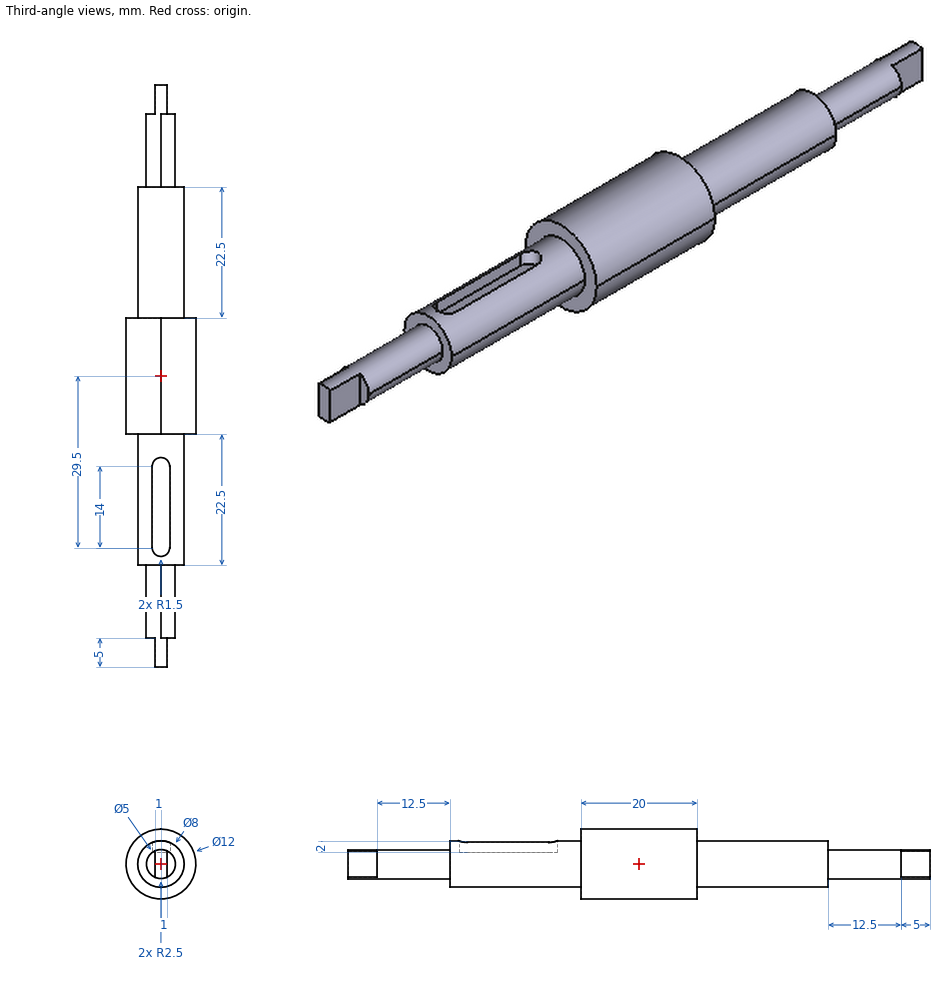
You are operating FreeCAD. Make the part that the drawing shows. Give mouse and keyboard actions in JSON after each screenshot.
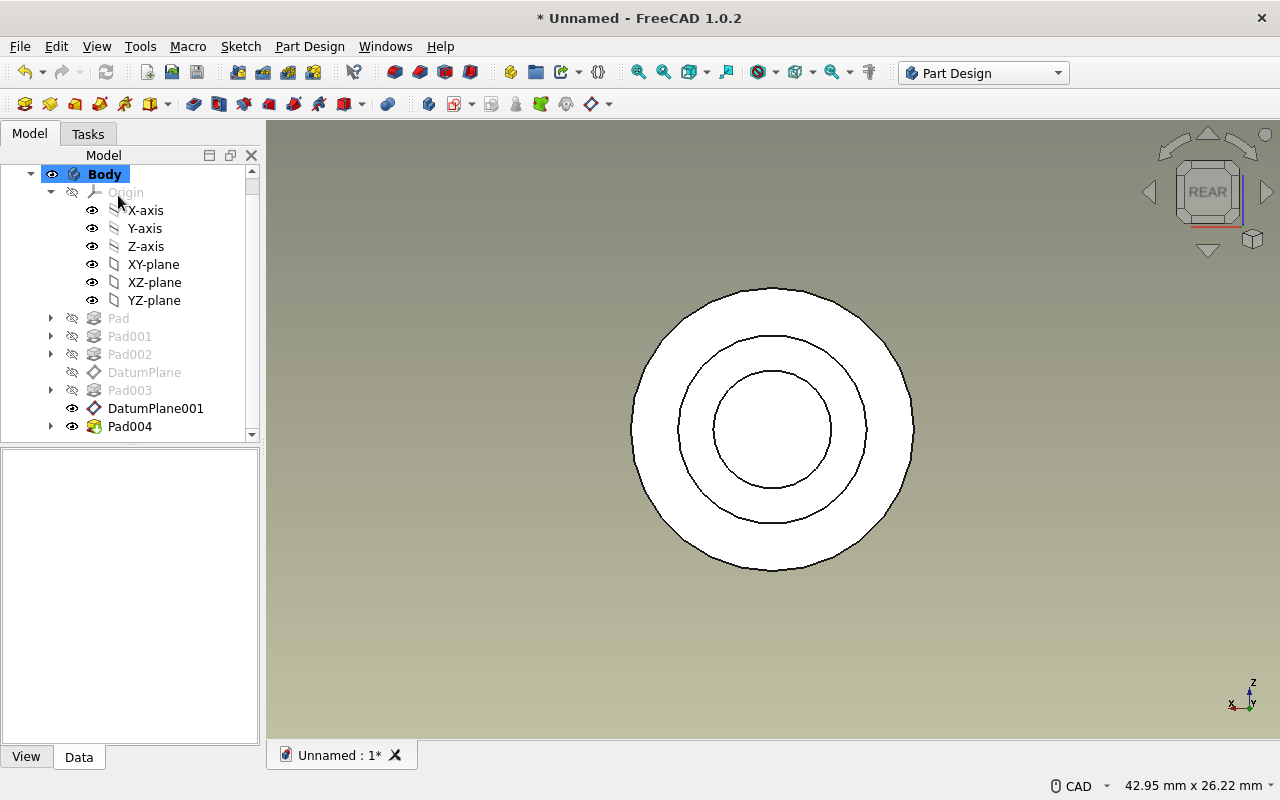
{"action": "left_click", "coordinate": [117, 408]}
{"action": "key", "text": "space"}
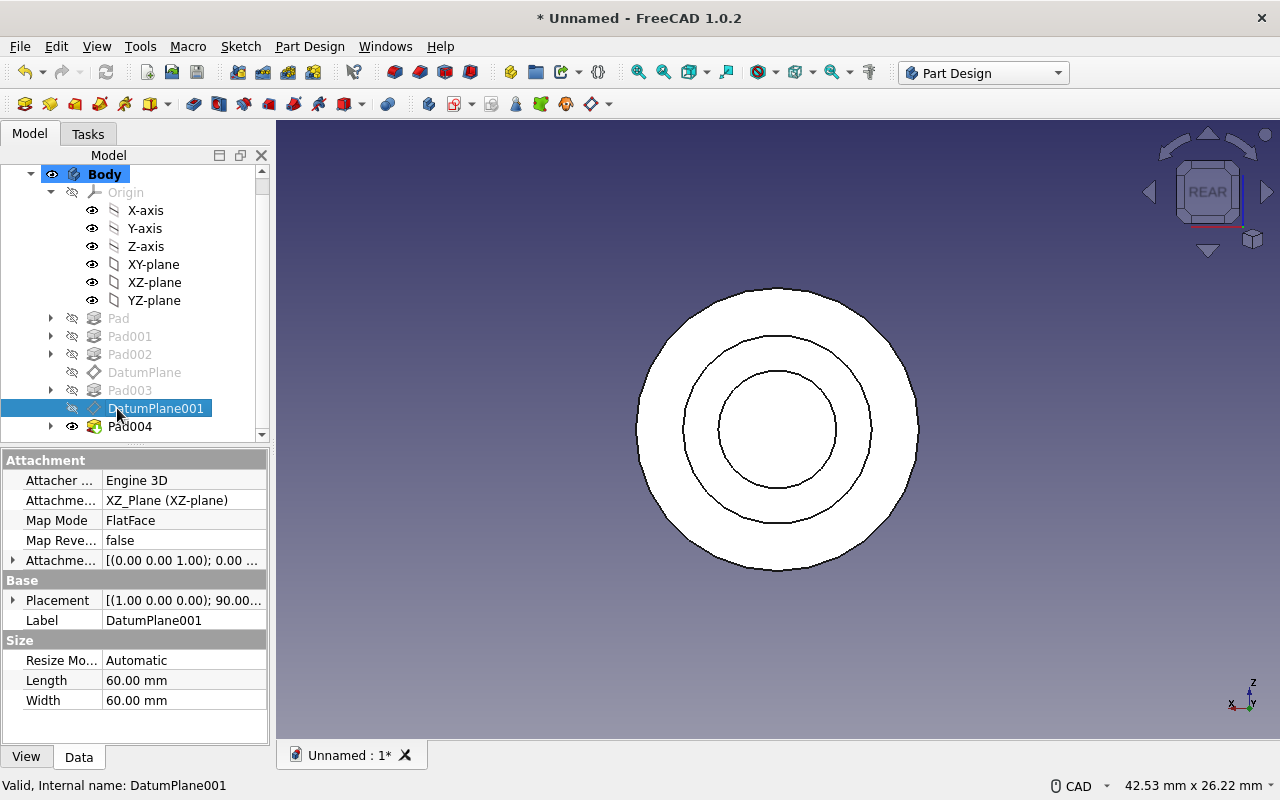
{"action": "left_click", "coordinate": [137, 282]}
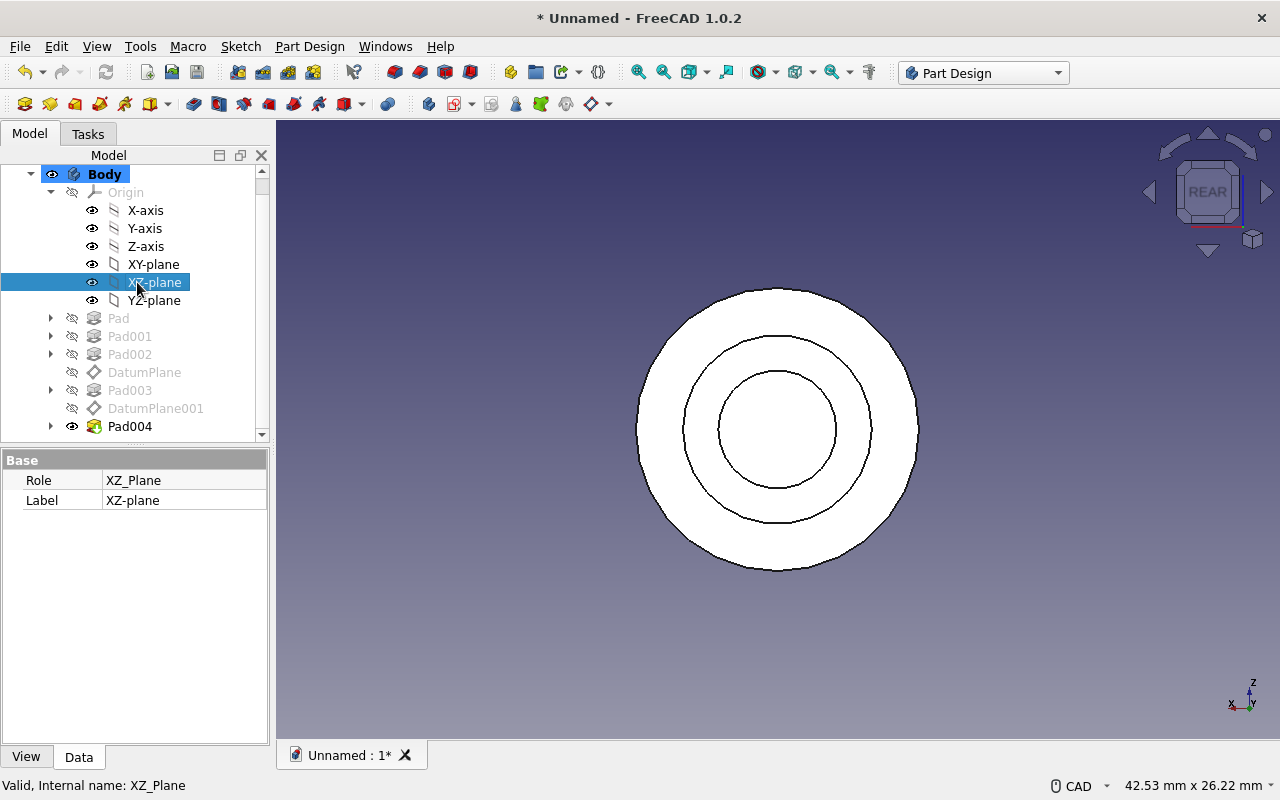
{"action": "left_click", "coordinate": [590, 104]}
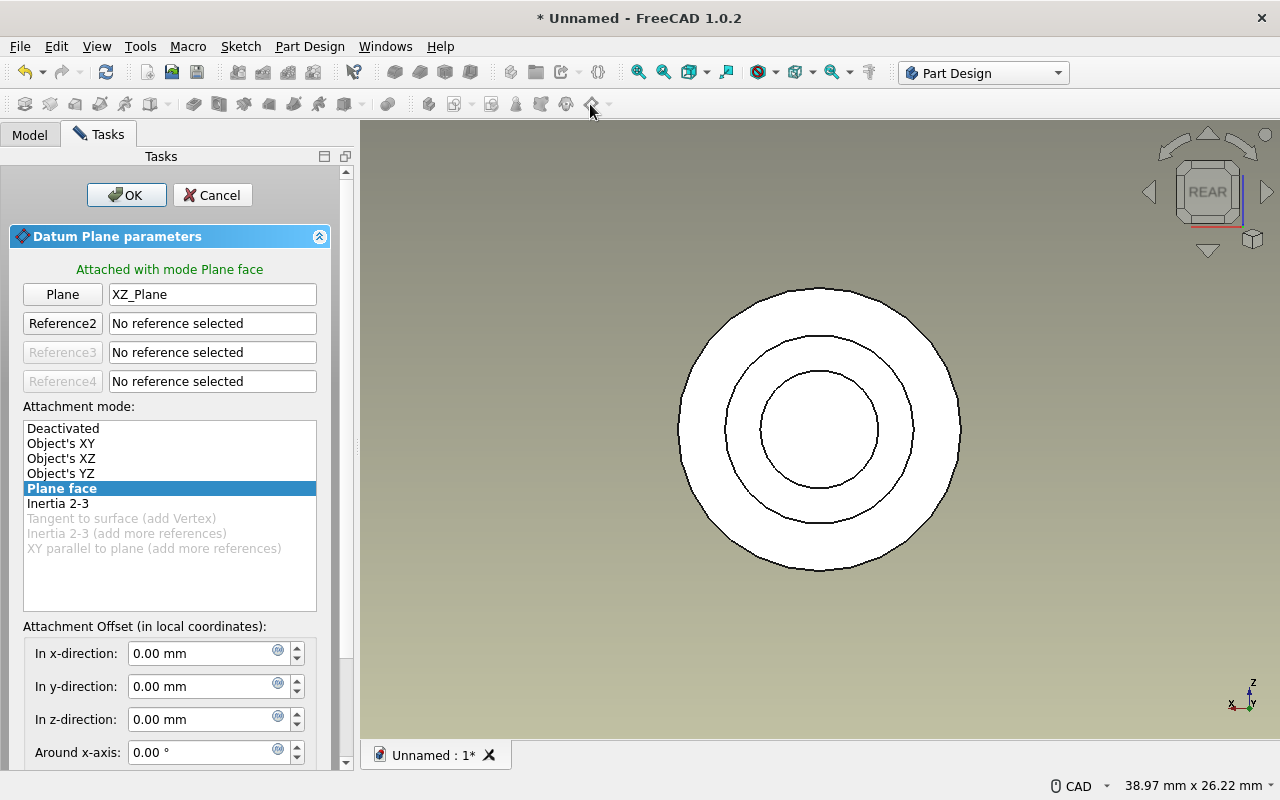
{"action": "triple_click", "coordinate": [210, 720]}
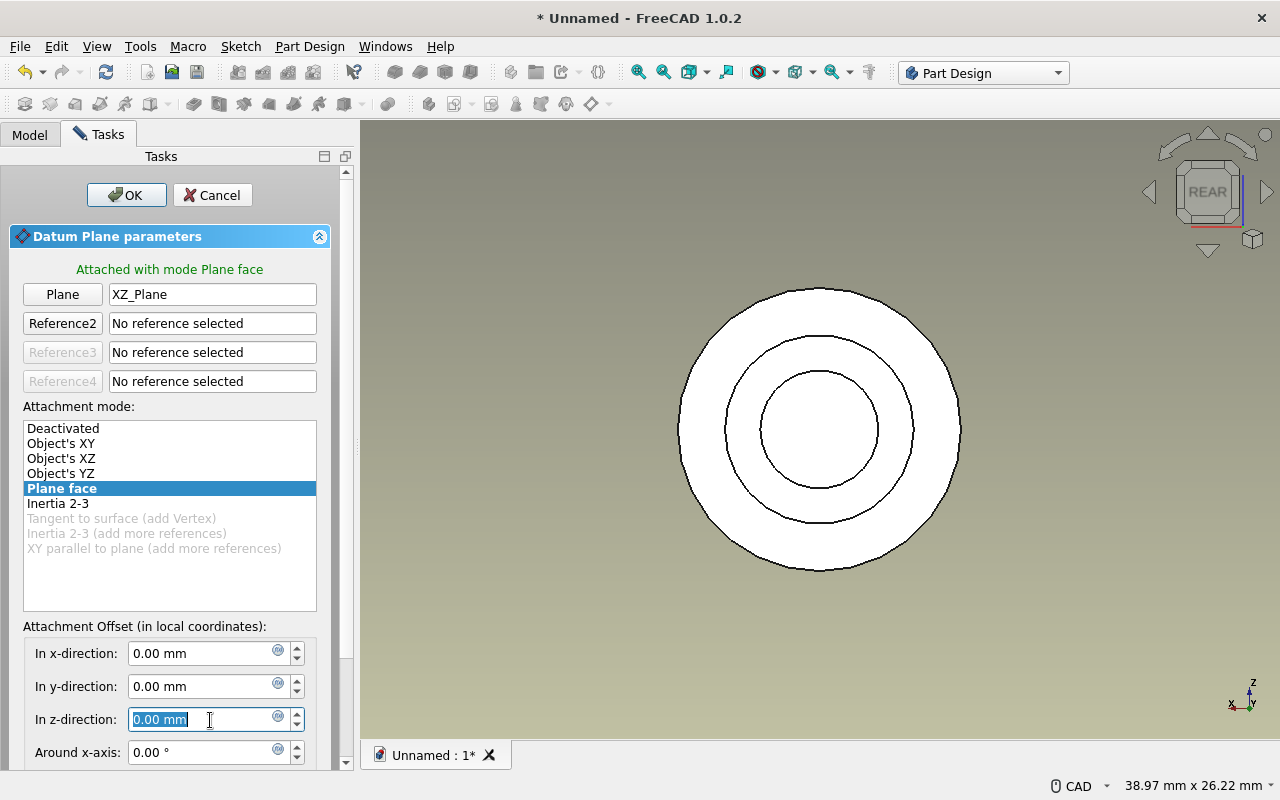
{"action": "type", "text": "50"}
{"action": "key", "text": "Tab"}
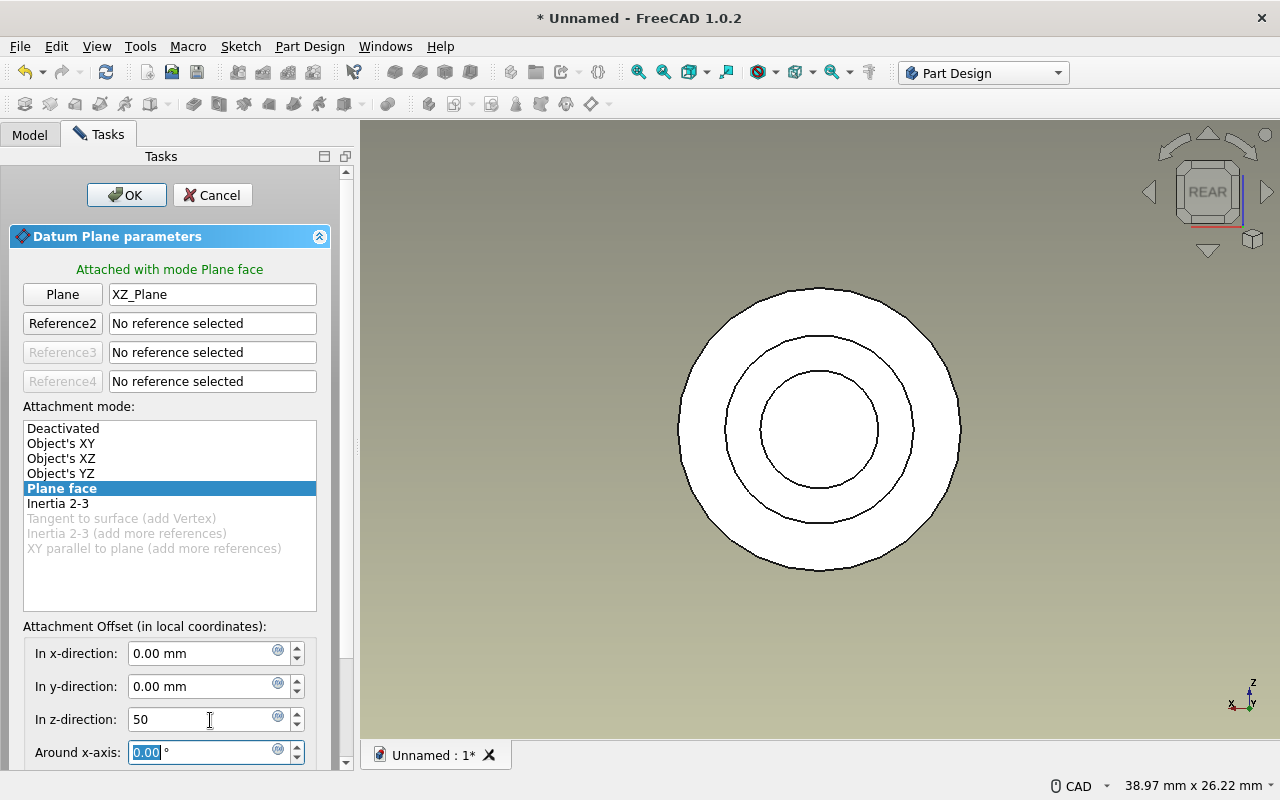
{"action": "left_click", "coordinate": [127, 195]}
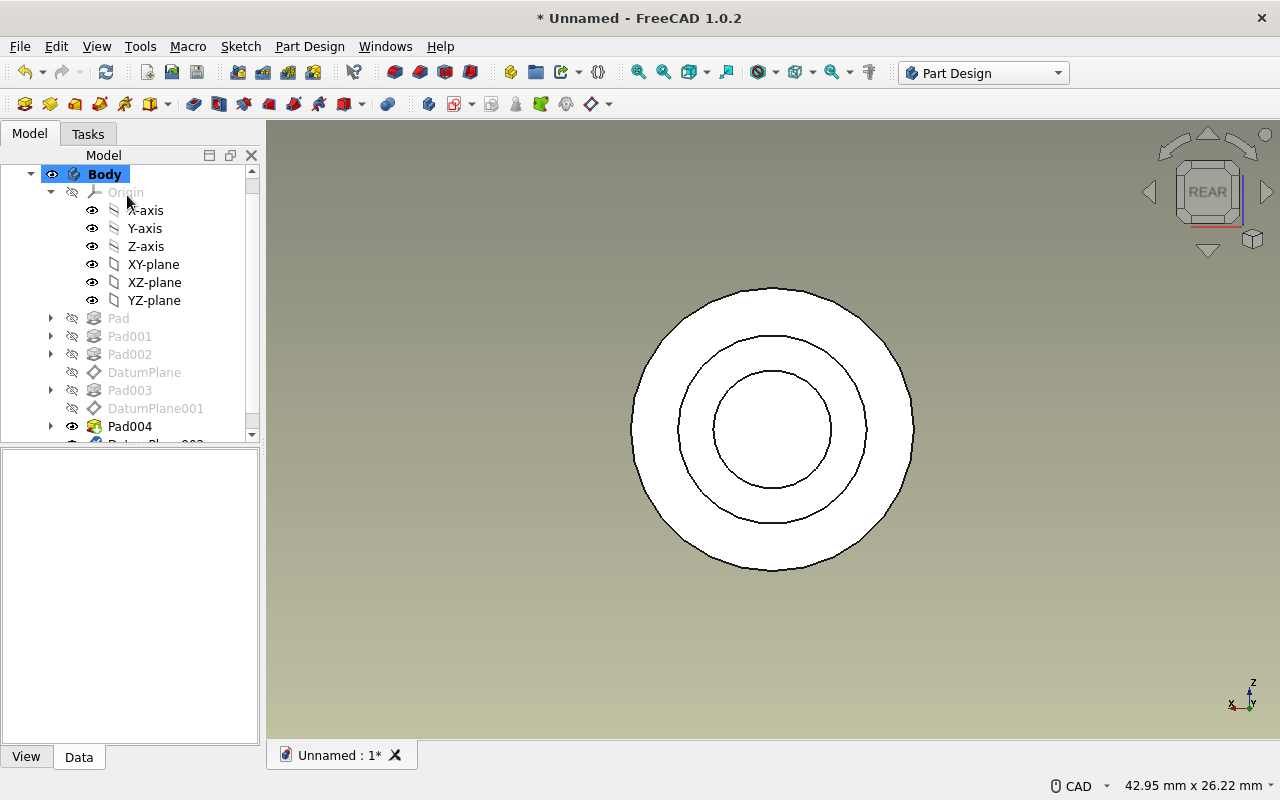
{"action": "scroll", "coordinate": [121, 296], "scroll_direction": "down", "scroll_amount": 3}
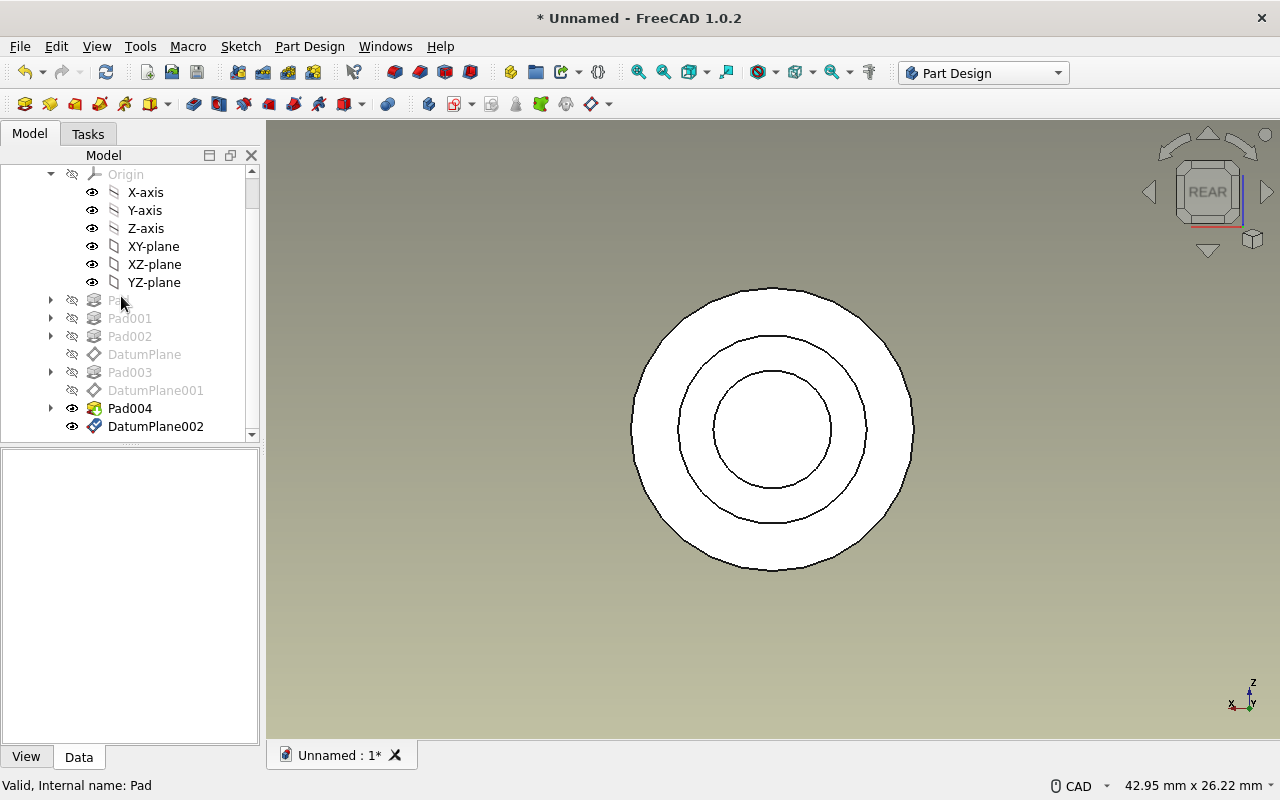
{"action": "left_click", "coordinate": [117, 426]}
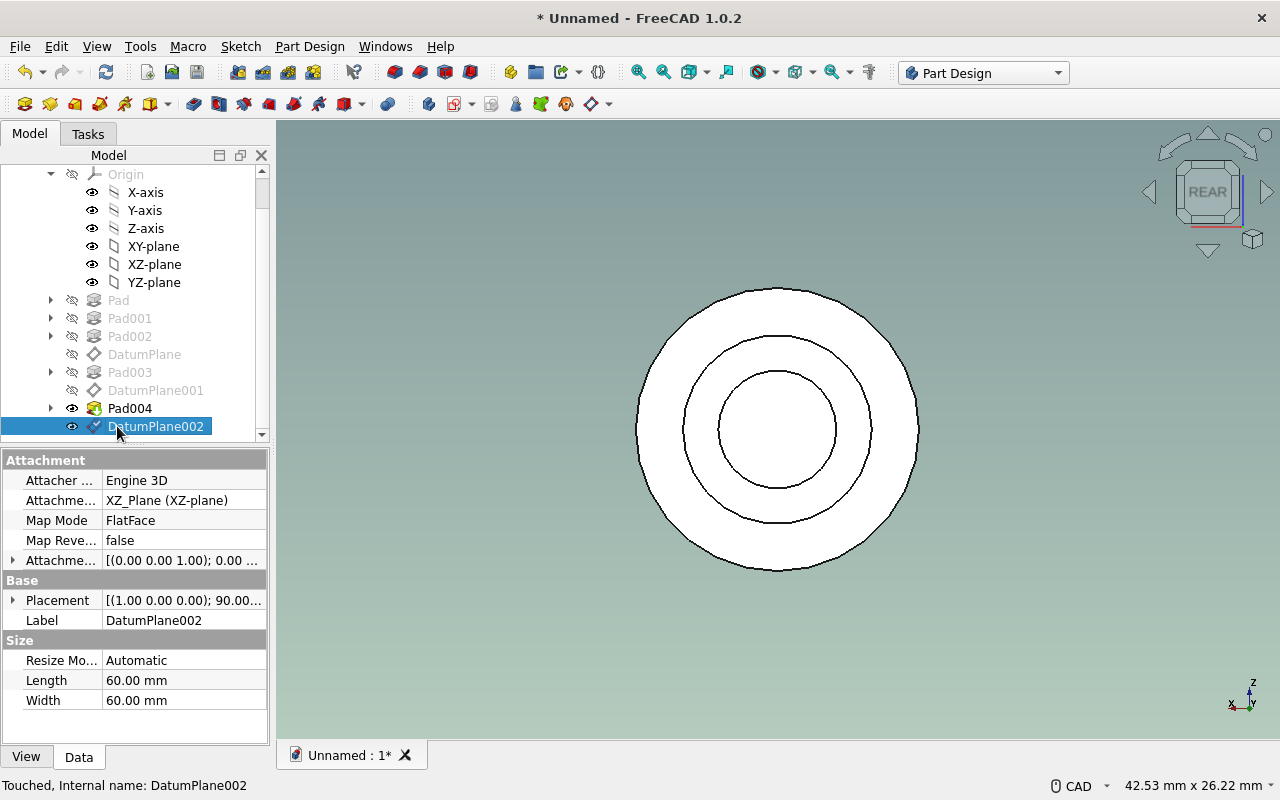
{"action": "left_click", "coordinate": [454, 104]}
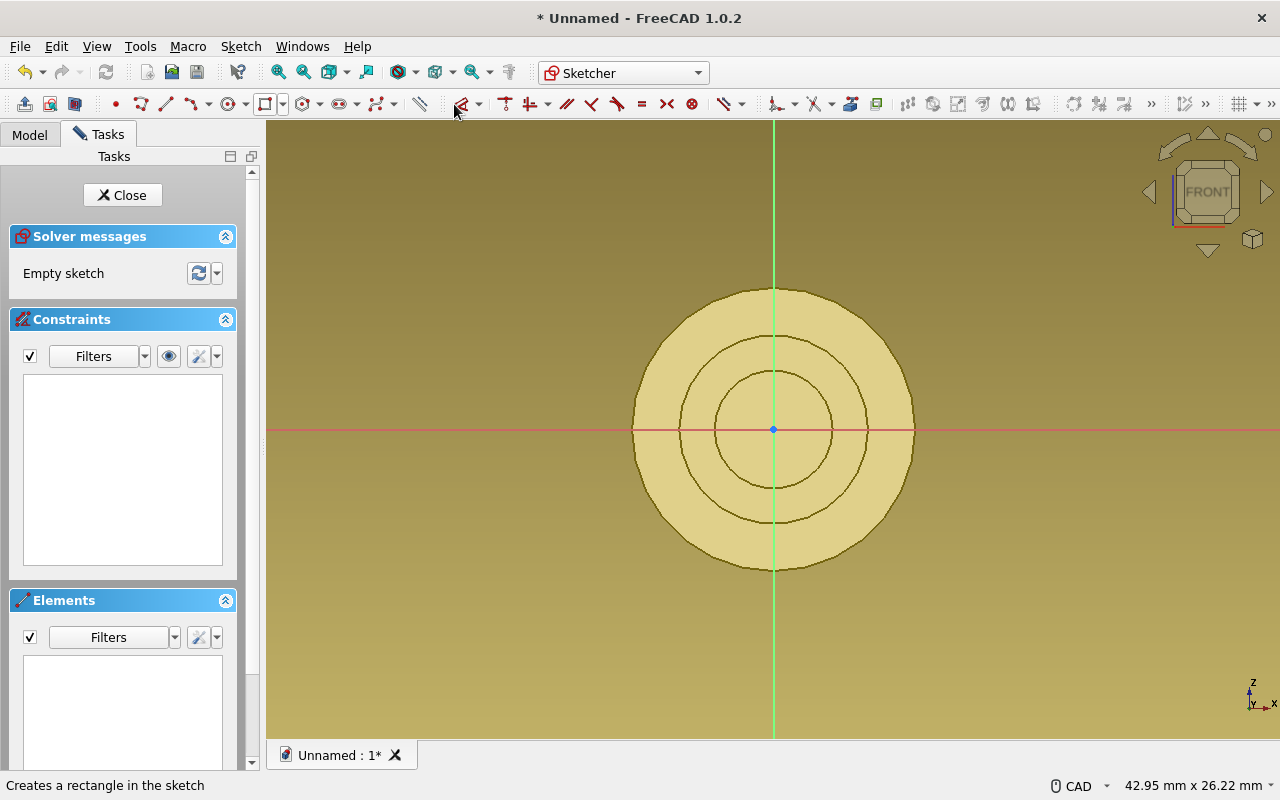
{"action": "scroll", "coordinate": [803, 429], "scroll_direction": "up", "scroll_amount": 6}